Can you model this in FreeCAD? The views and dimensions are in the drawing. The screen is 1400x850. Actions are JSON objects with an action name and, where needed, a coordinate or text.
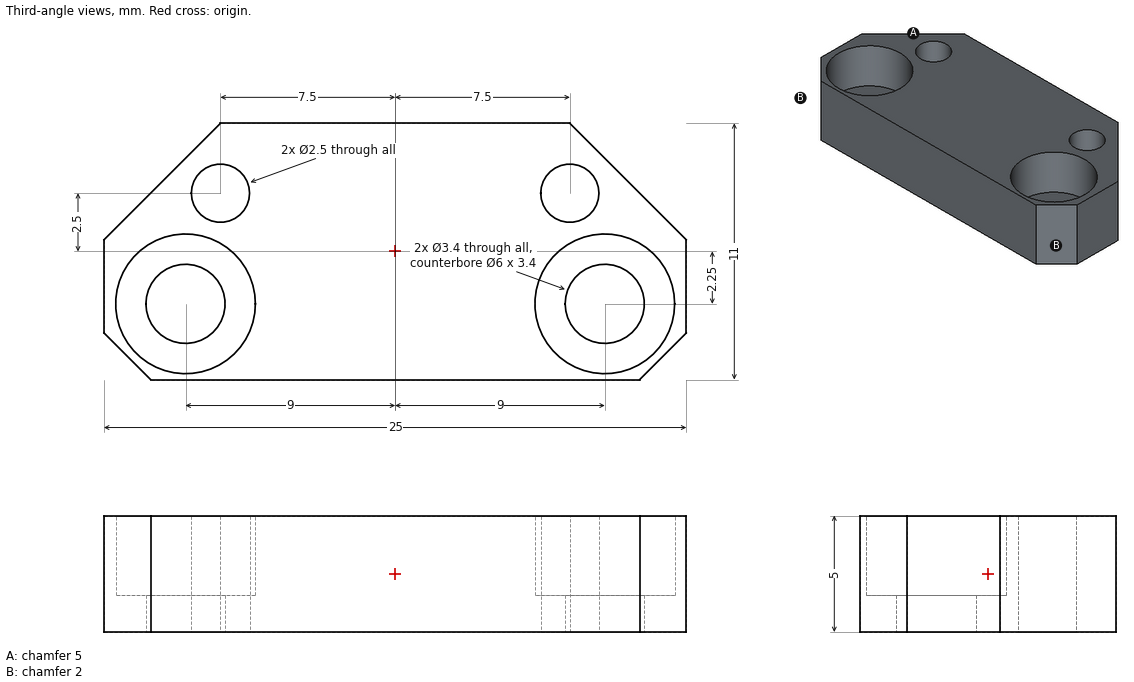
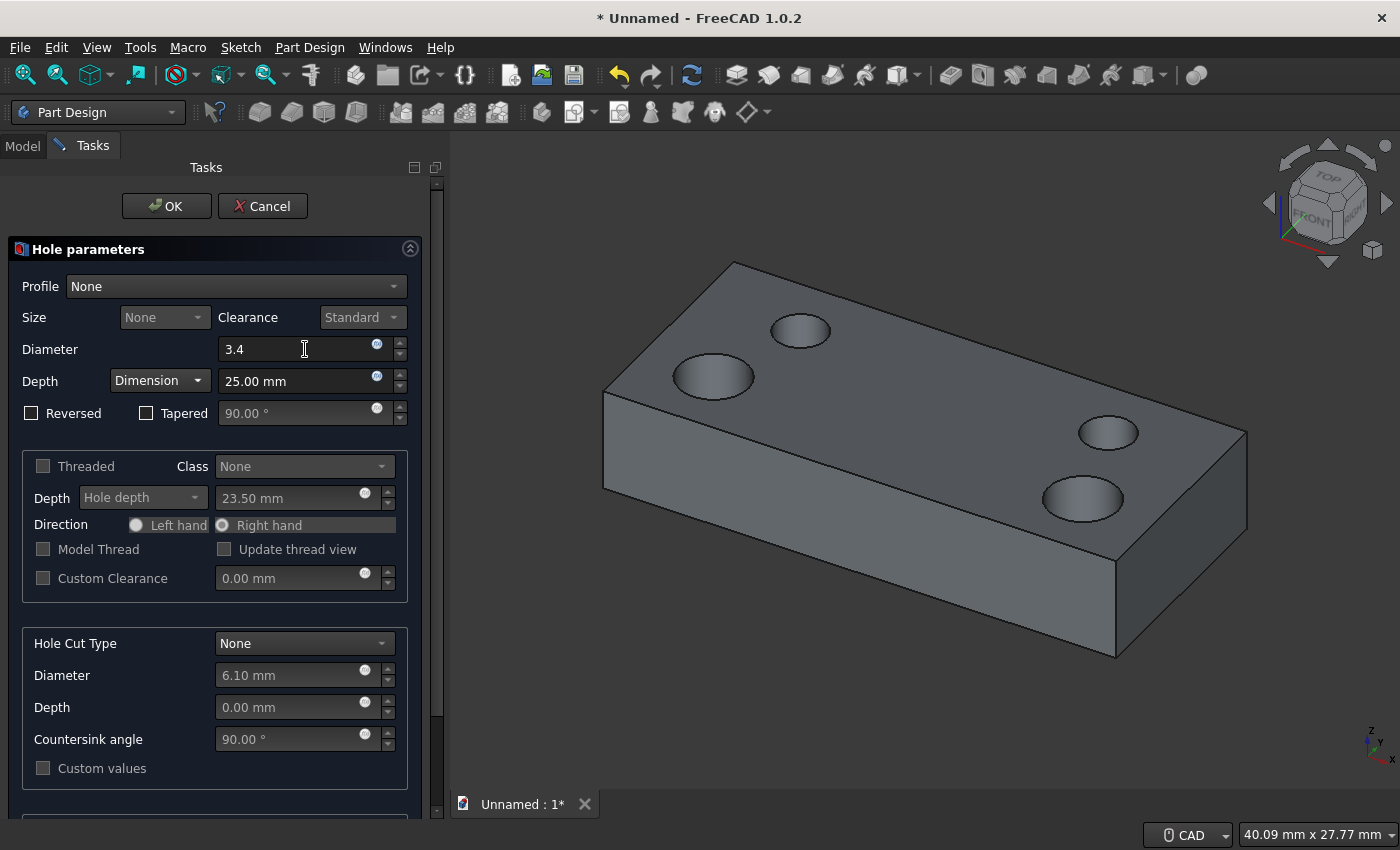
{"action": "left_click", "coordinate": [161, 380]}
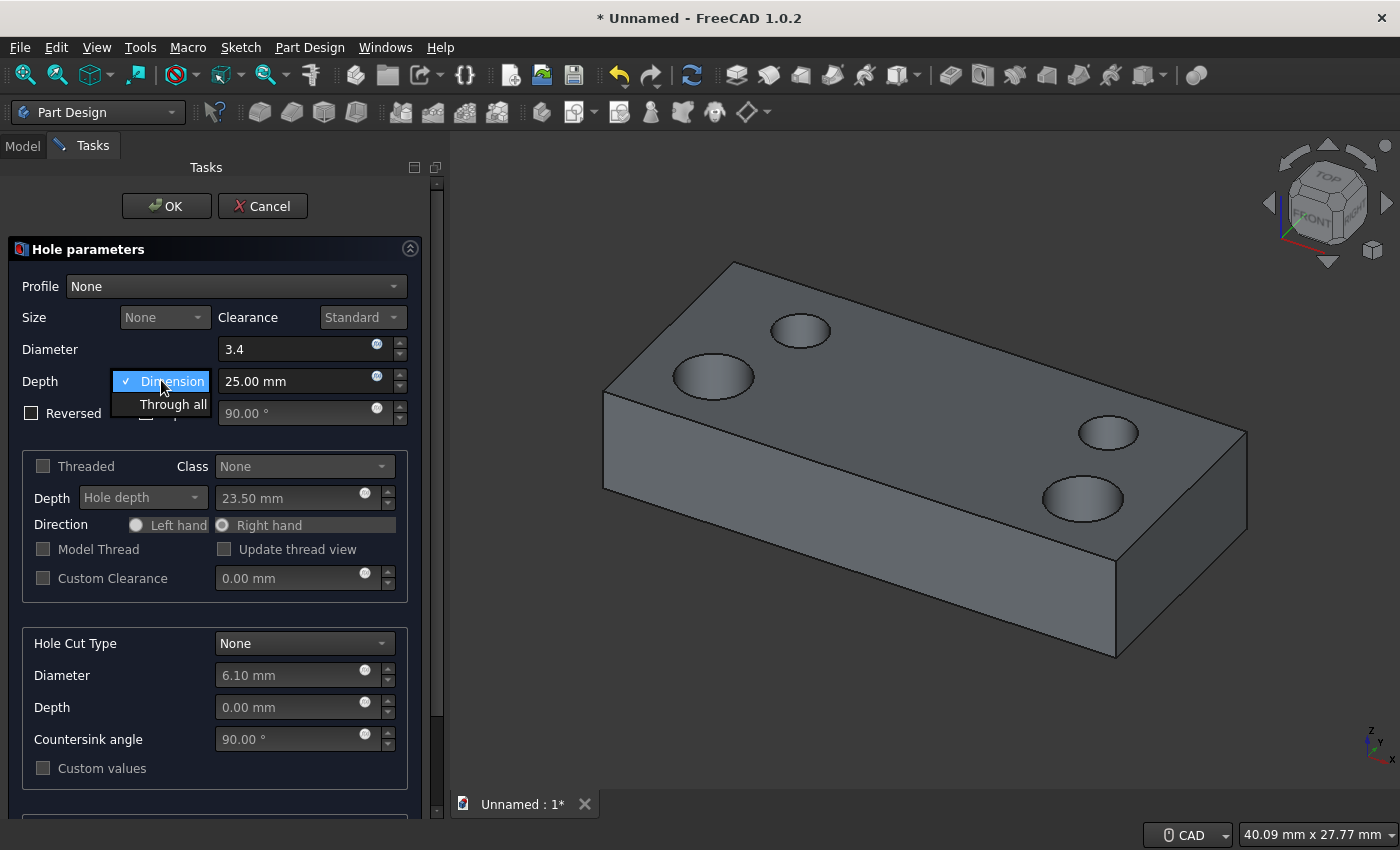
{"action": "left_click", "coordinate": [160, 404]}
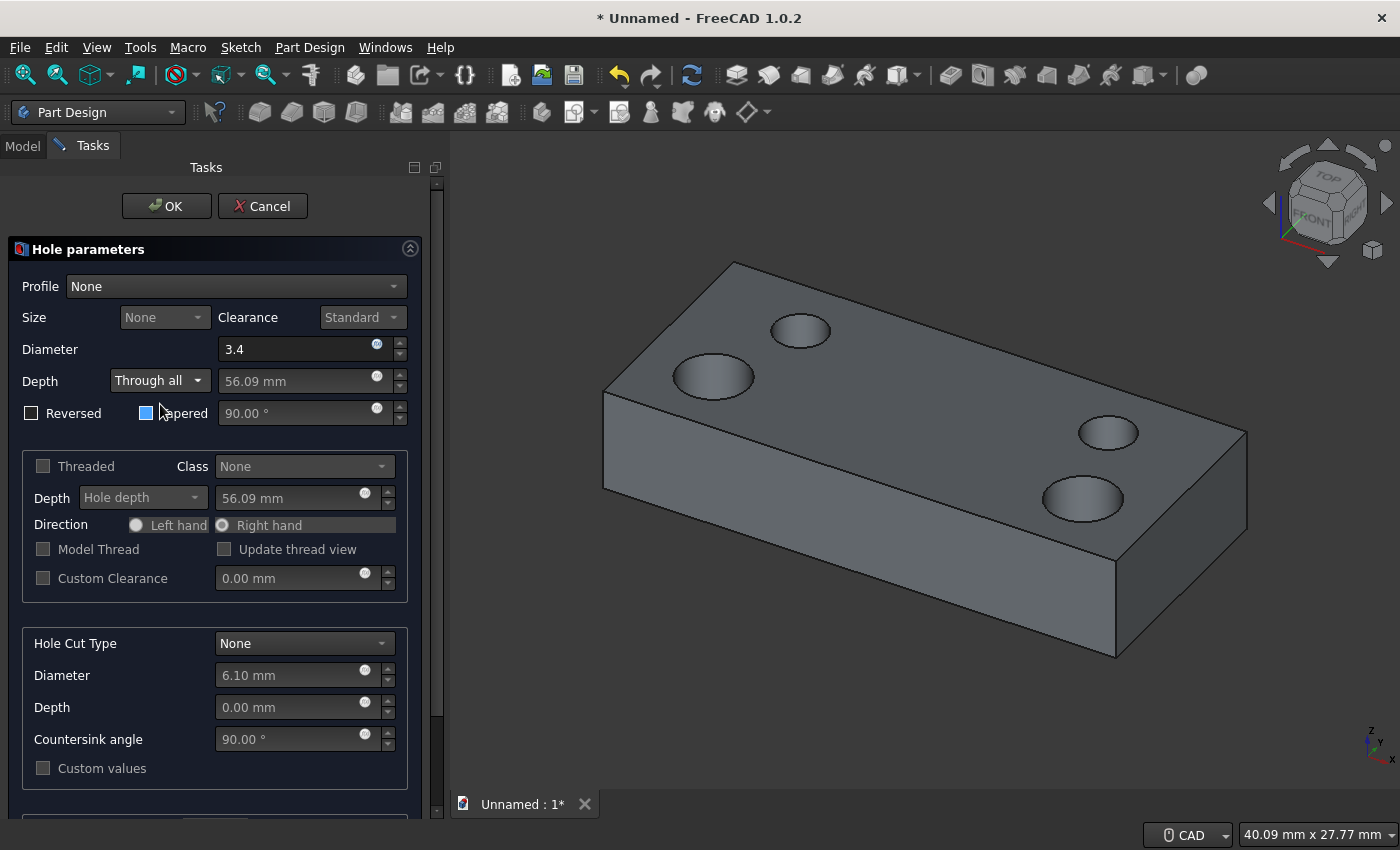
{"action": "left_click", "coordinate": [306, 644]}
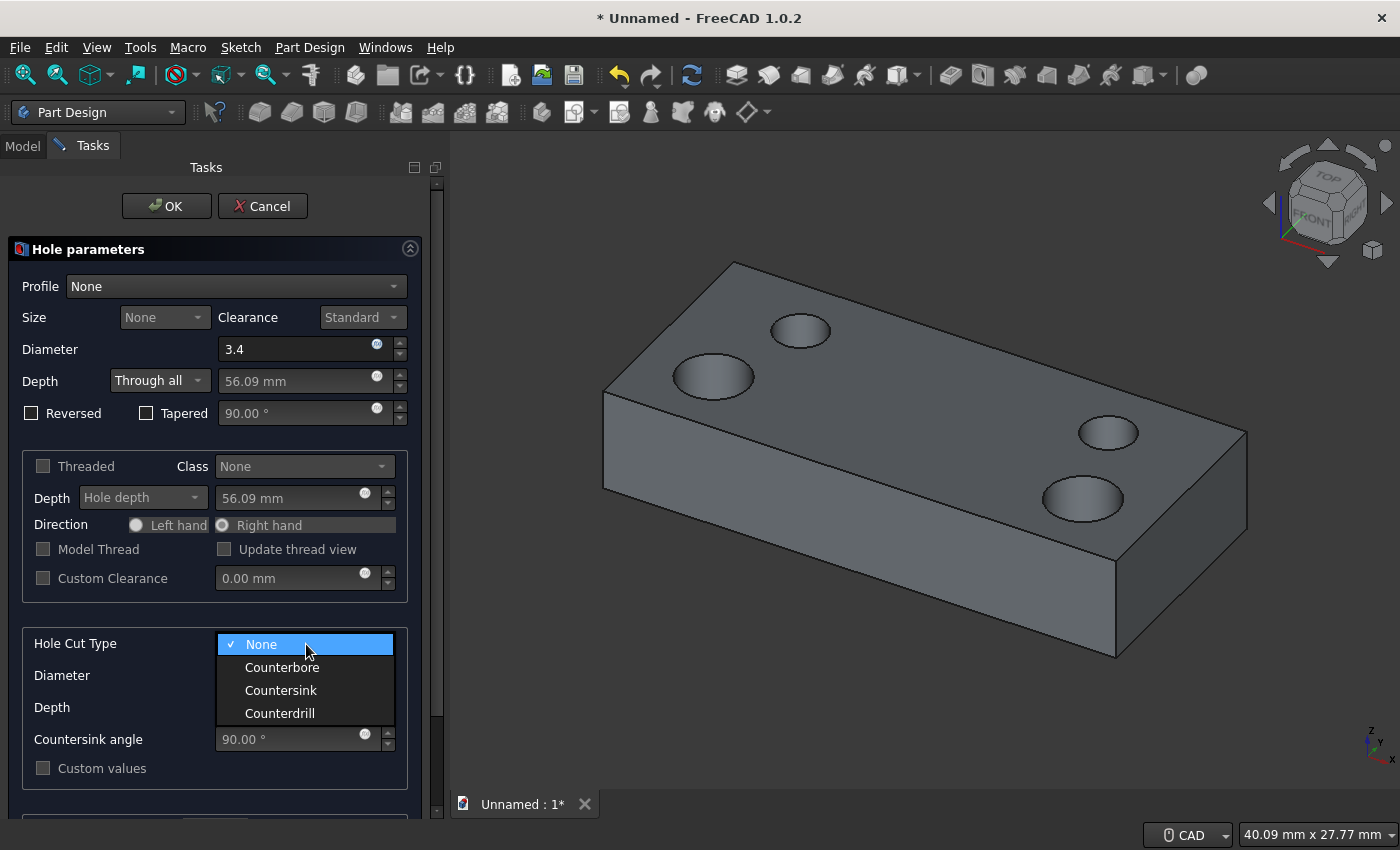
{"action": "left_click", "coordinate": [304, 668]}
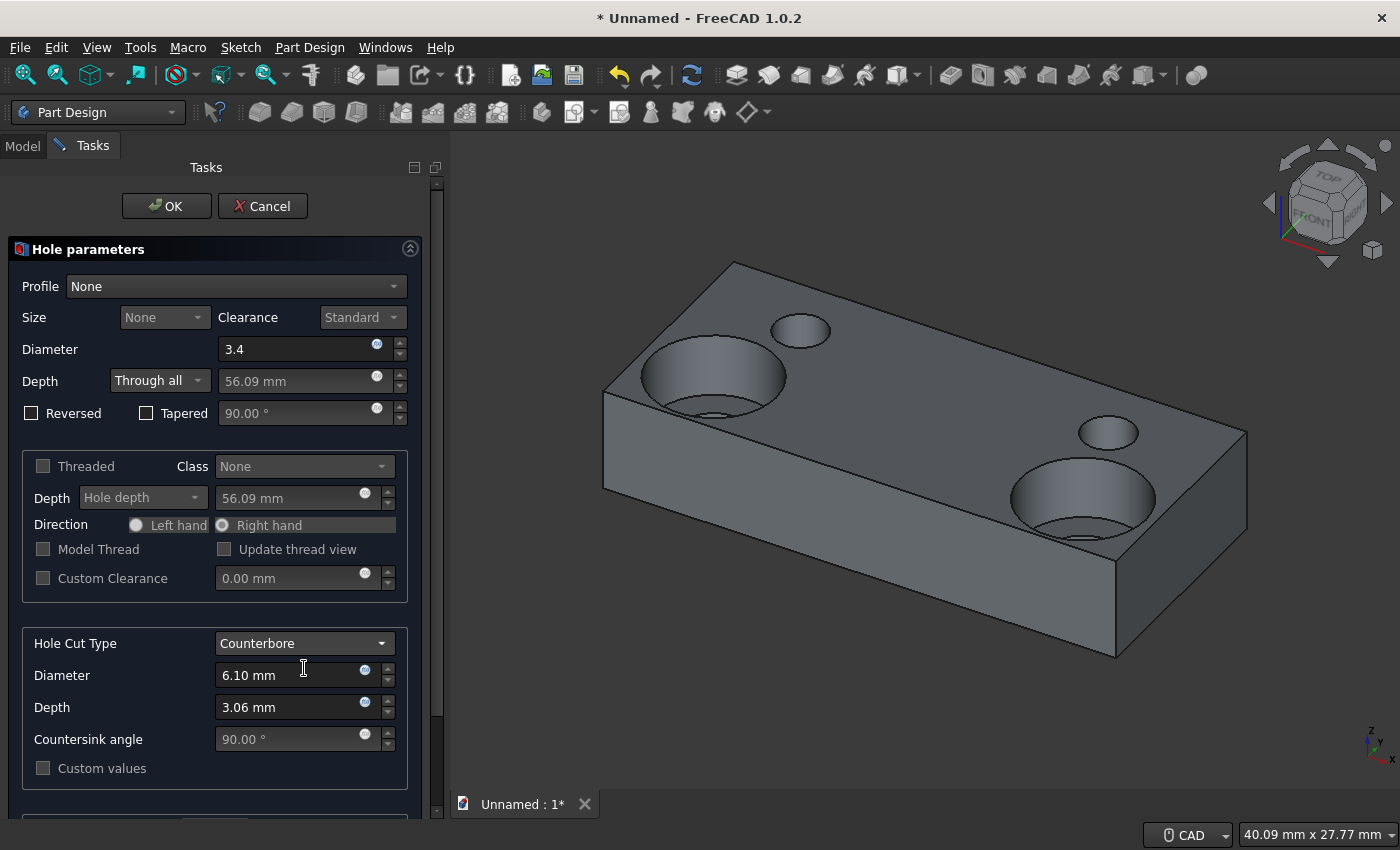
{"action": "triple_click", "coordinate": [298, 675]}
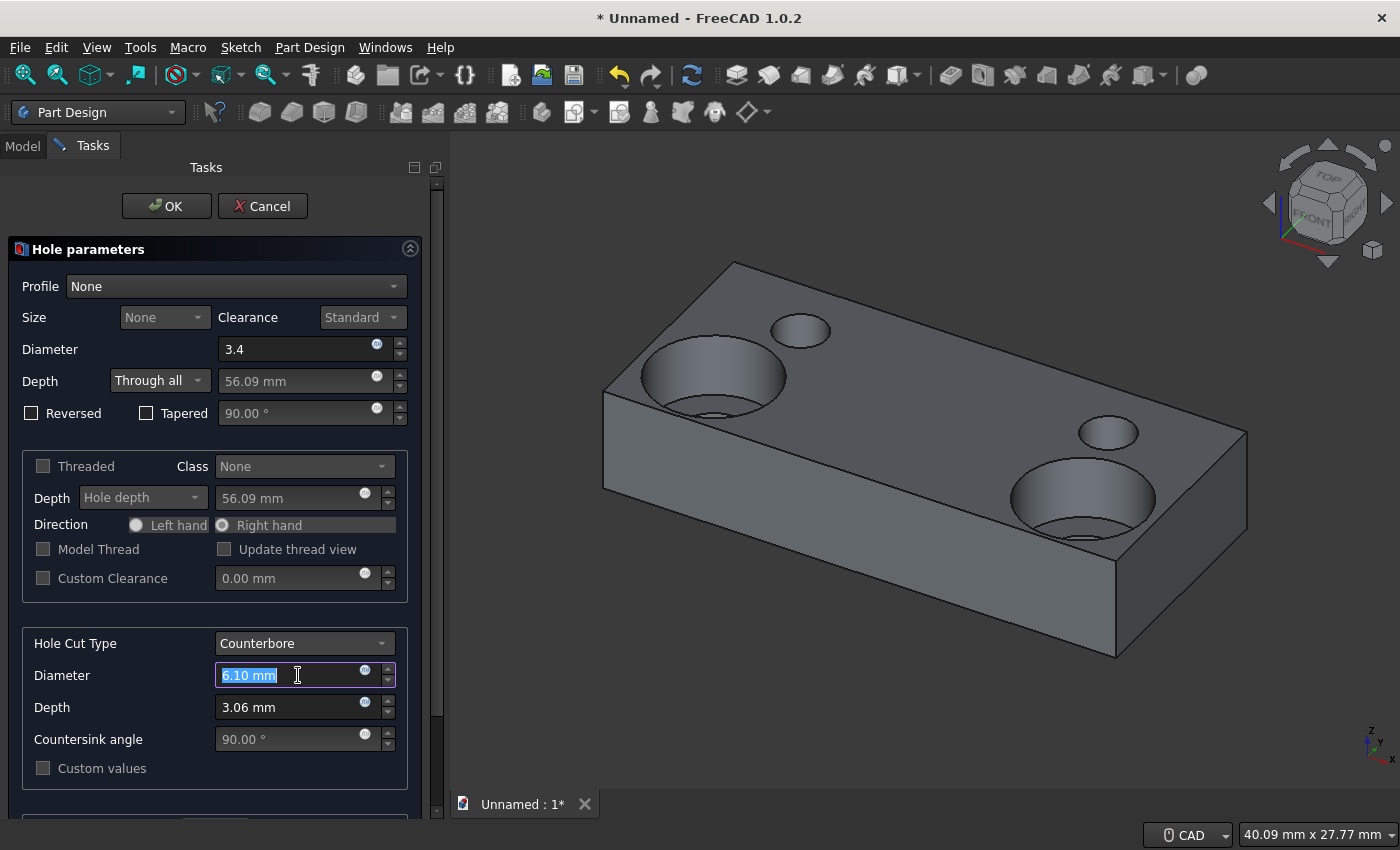
{"action": "type", "text": "6"}
{"action": "key", "text": "Tab"}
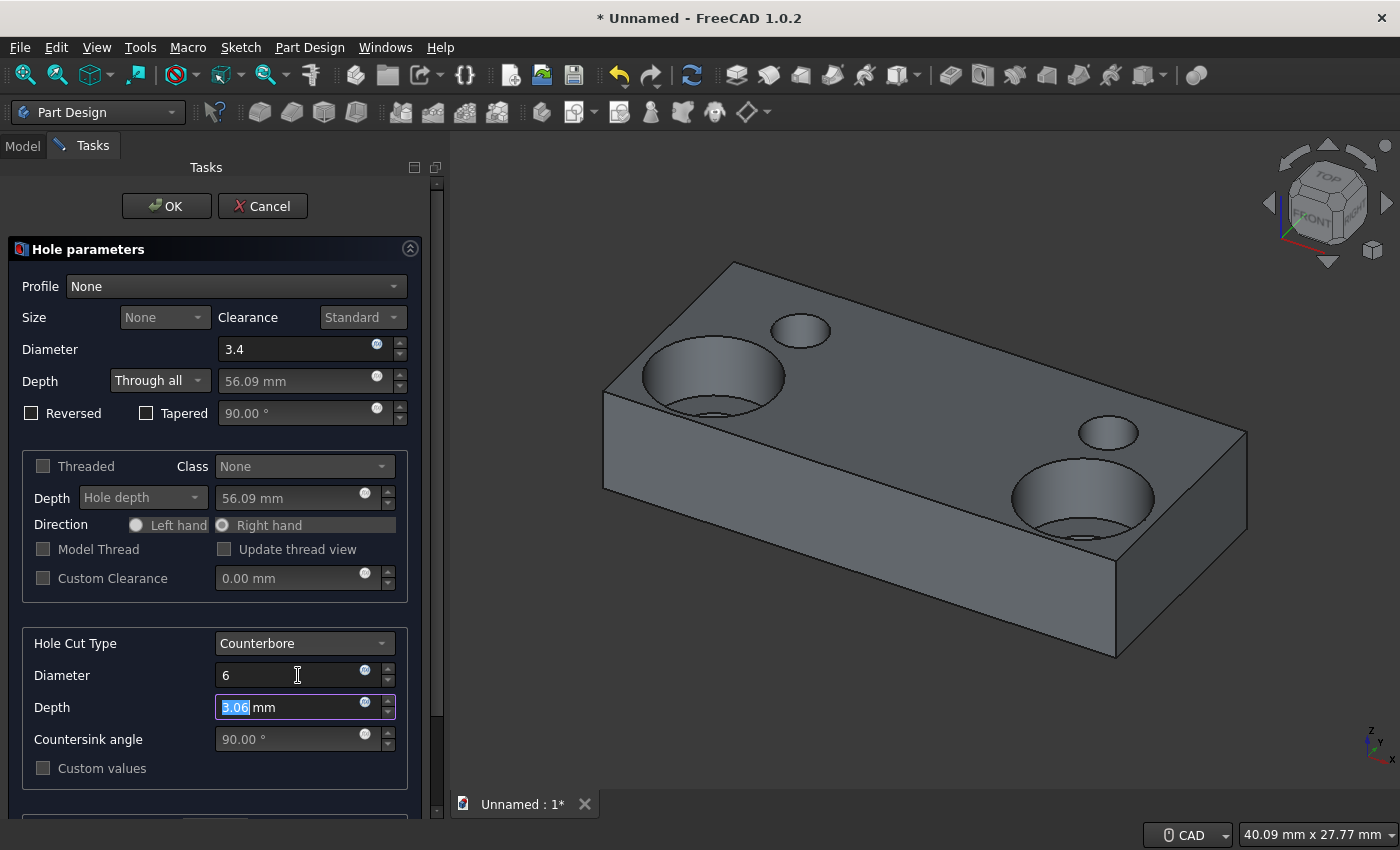
{"action": "type", "text": "3.4"}
{"action": "key", "text": "Tab"}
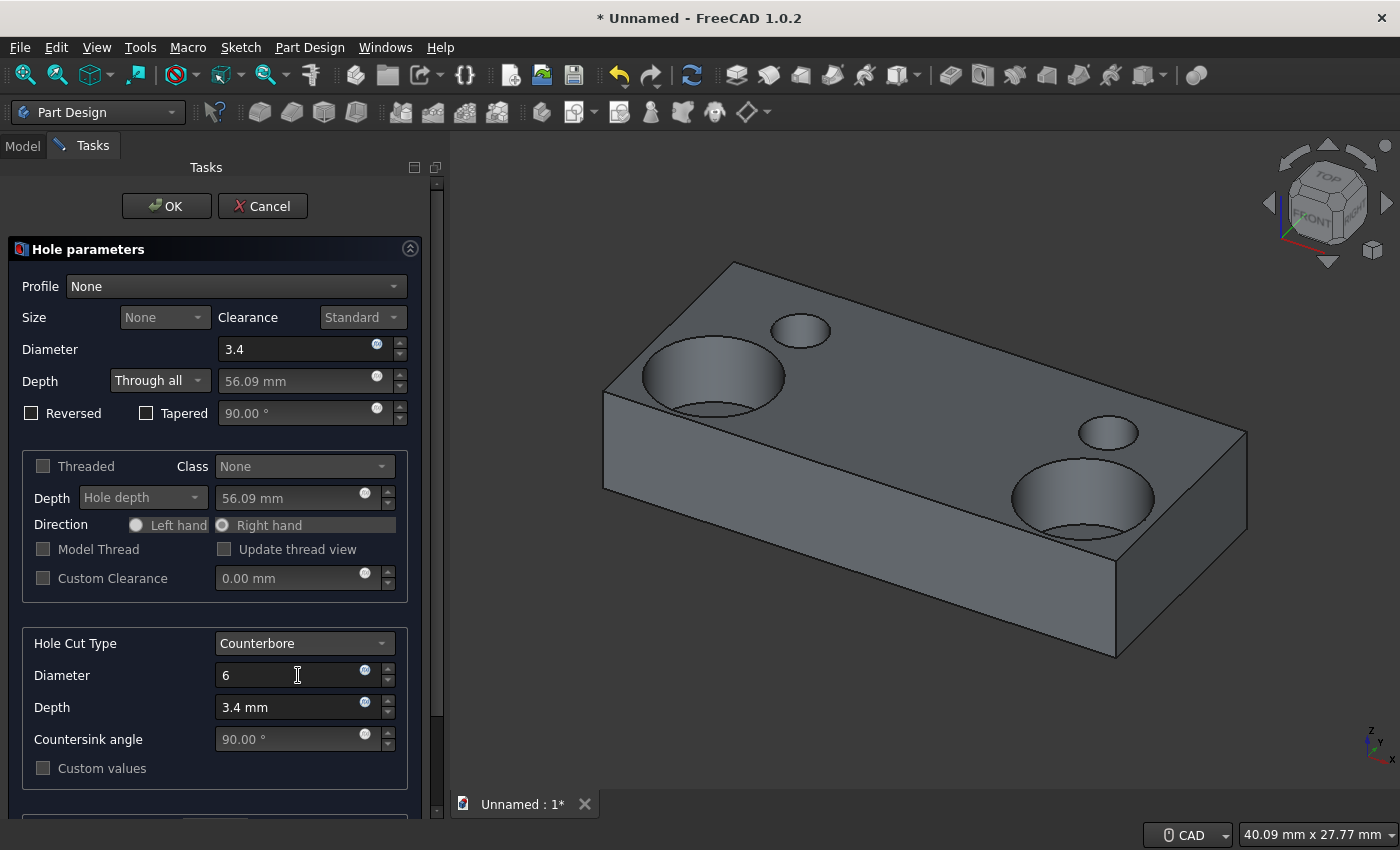
{"action": "left_click", "coordinate": [167, 206]}